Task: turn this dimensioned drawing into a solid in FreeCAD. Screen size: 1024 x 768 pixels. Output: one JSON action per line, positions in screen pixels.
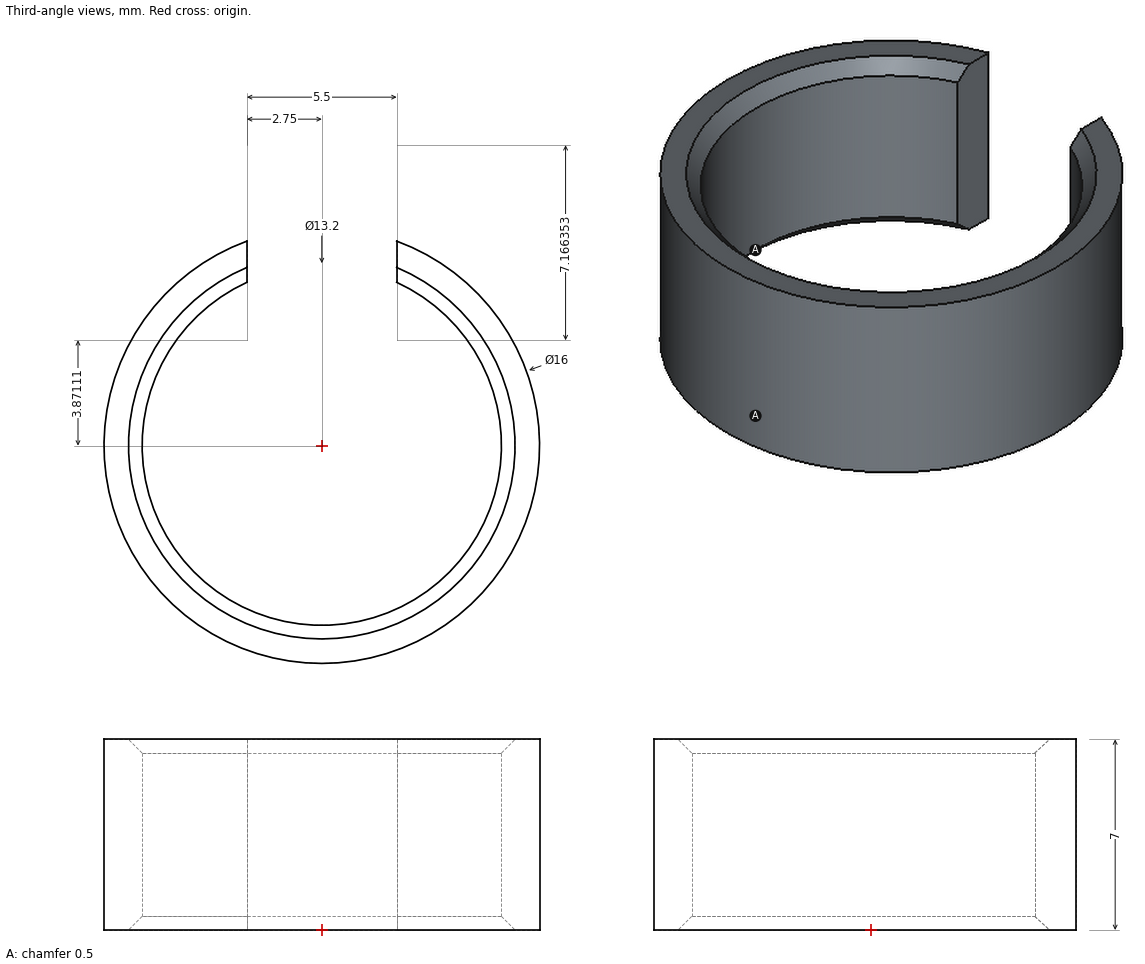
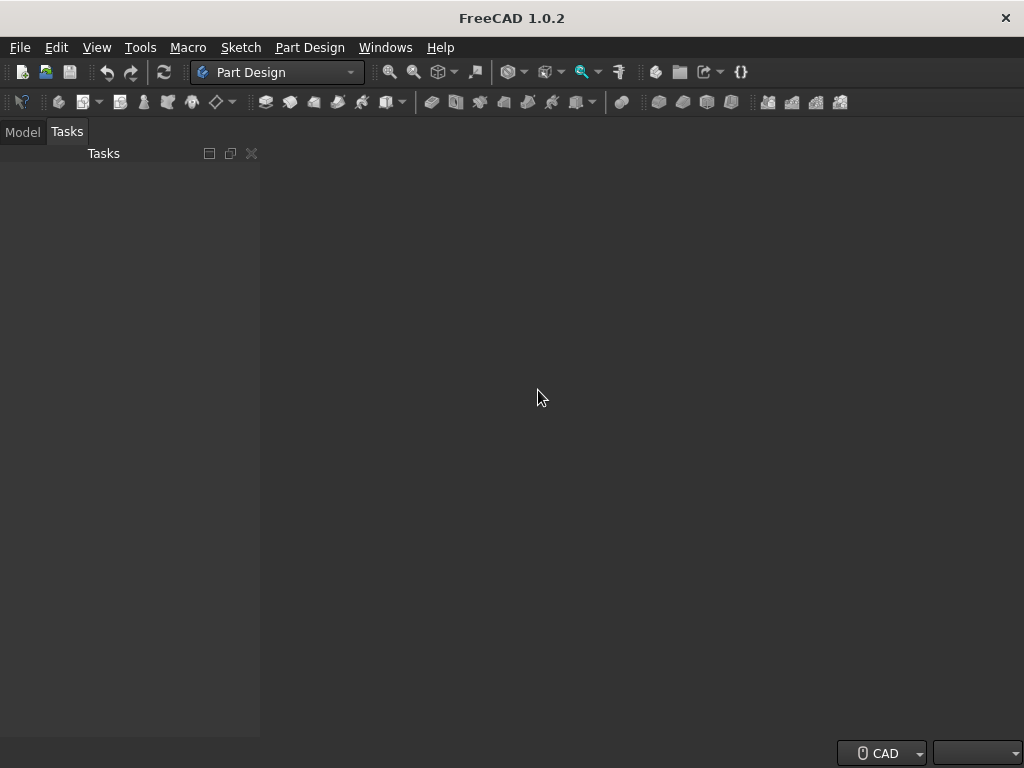
{"action": "left_click", "coordinate": [22, 72]}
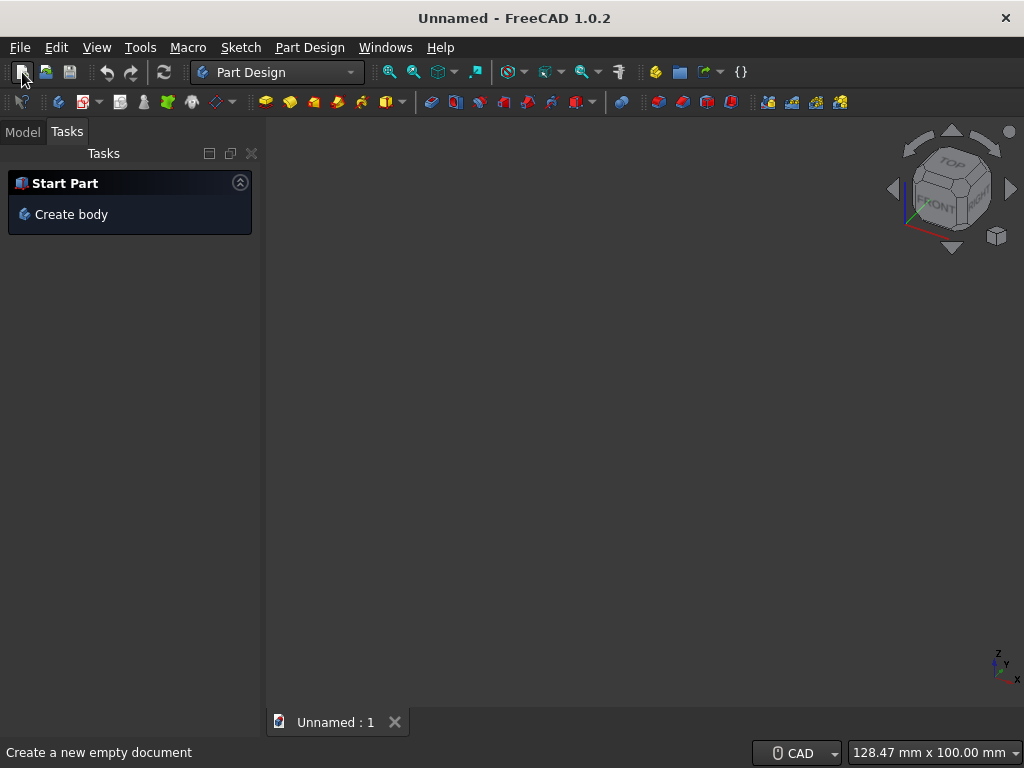
{"action": "left_click", "coordinate": [84, 102]}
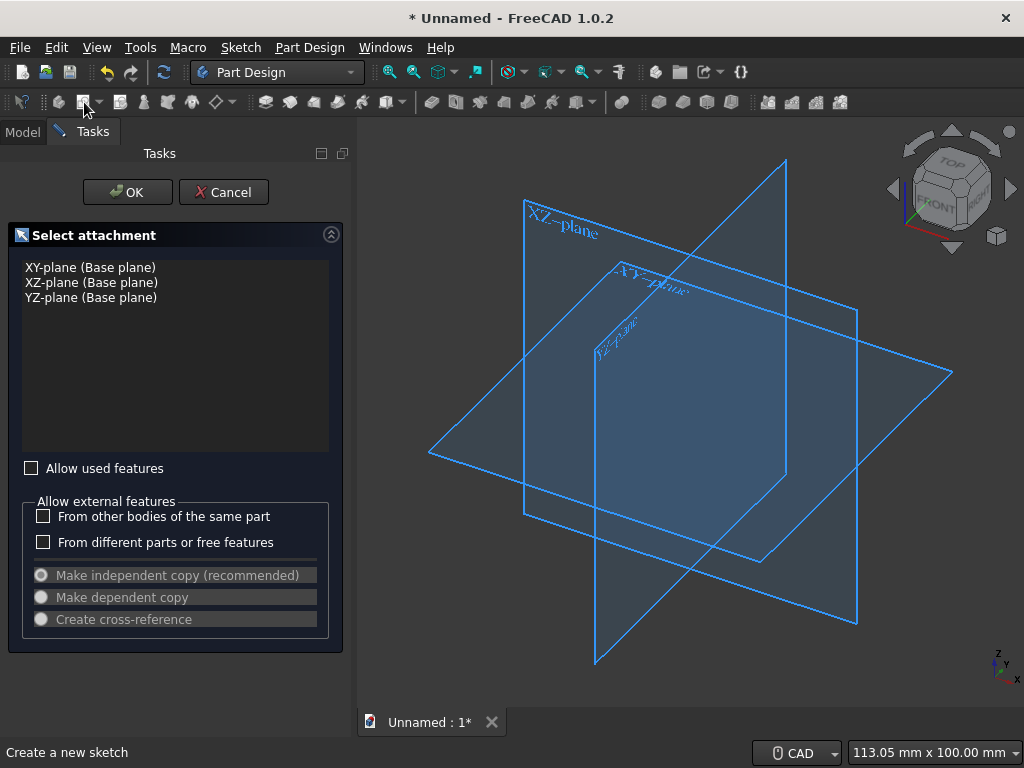
{"action": "left_click", "coordinate": [82, 268]}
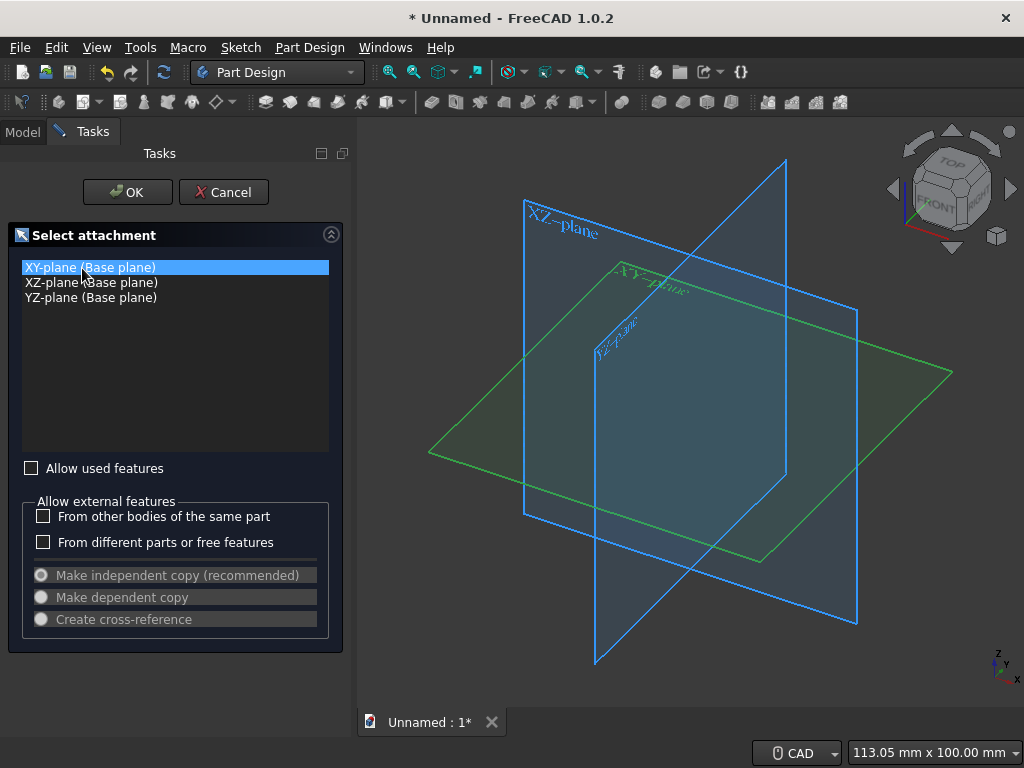
{"action": "left_click", "coordinate": [128, 192]}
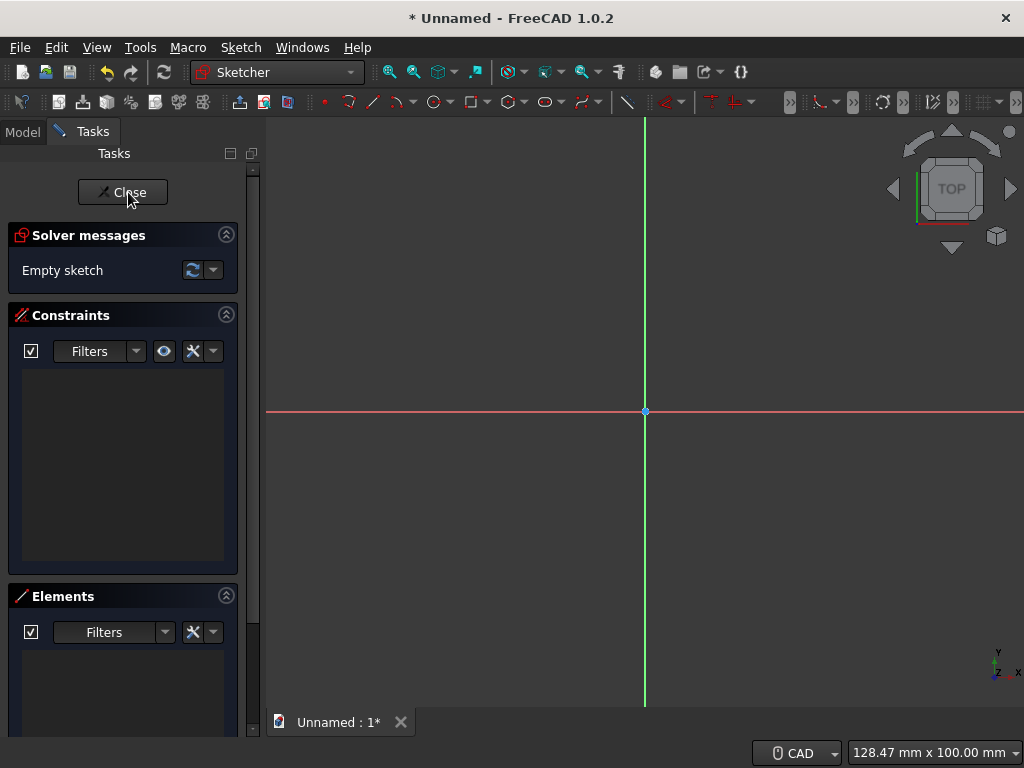
{"action": "scroll", "coordinate": [667, 412], "scroll_direction": "up", "scroll_amount": 7}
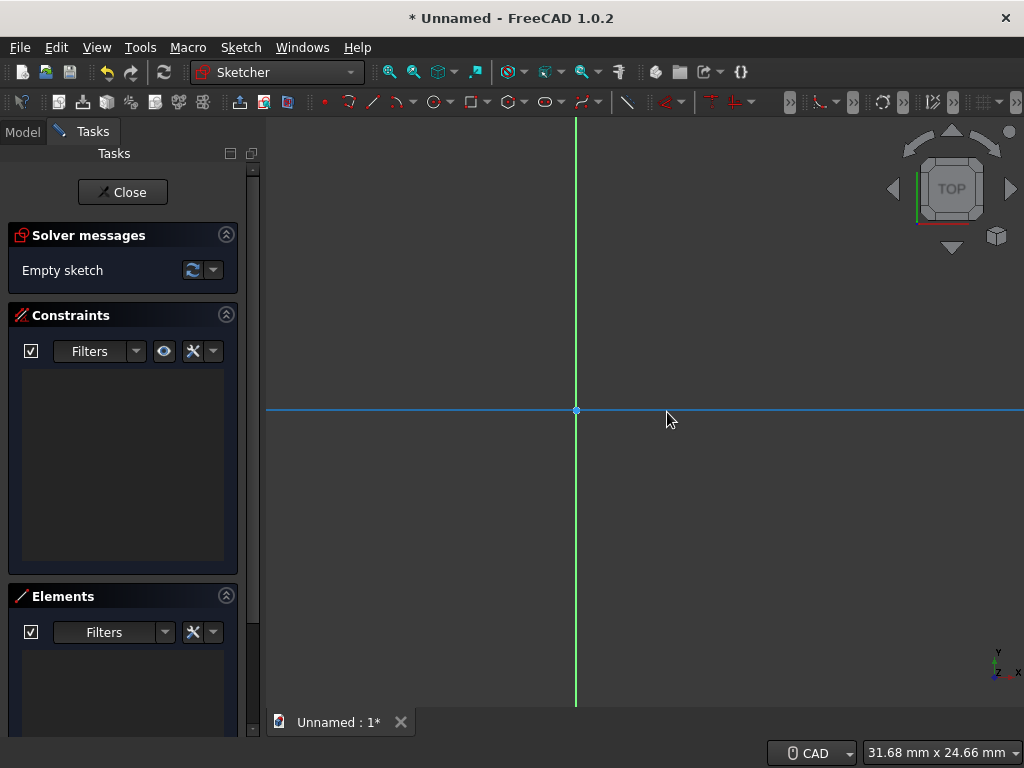
{"action": "left_click", "coordinate": [434, 102]}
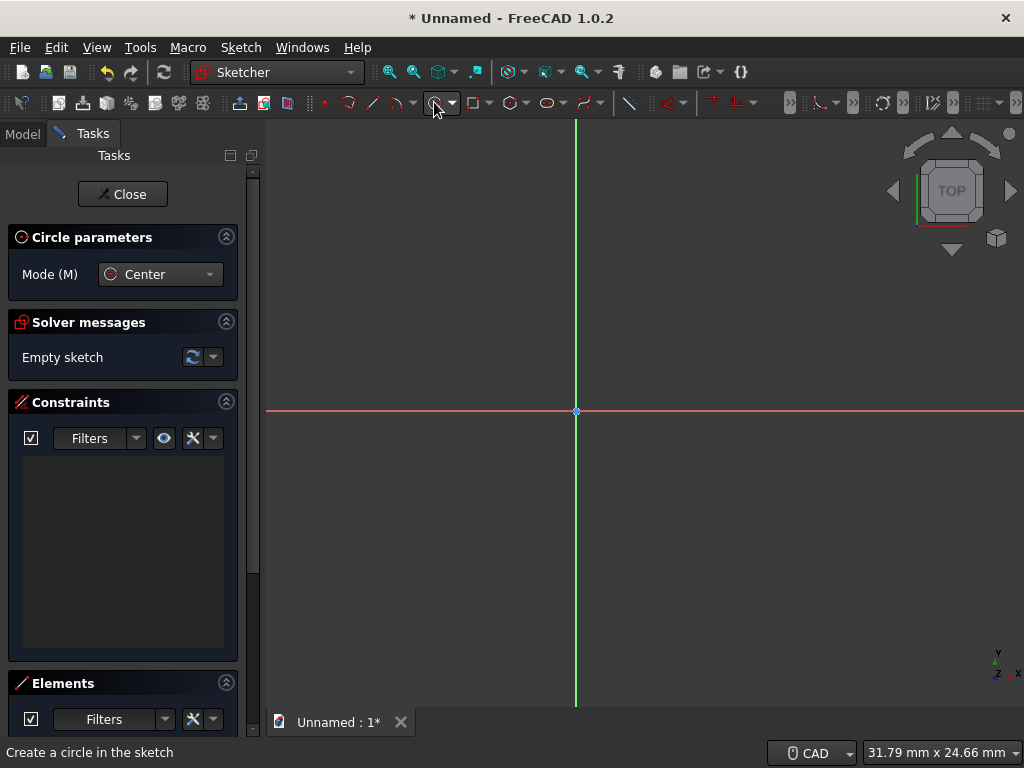
{"action": "left_click", "coordinate": [576, 411]}
{"action": "mouse_move", "coordinate": [711, 277]}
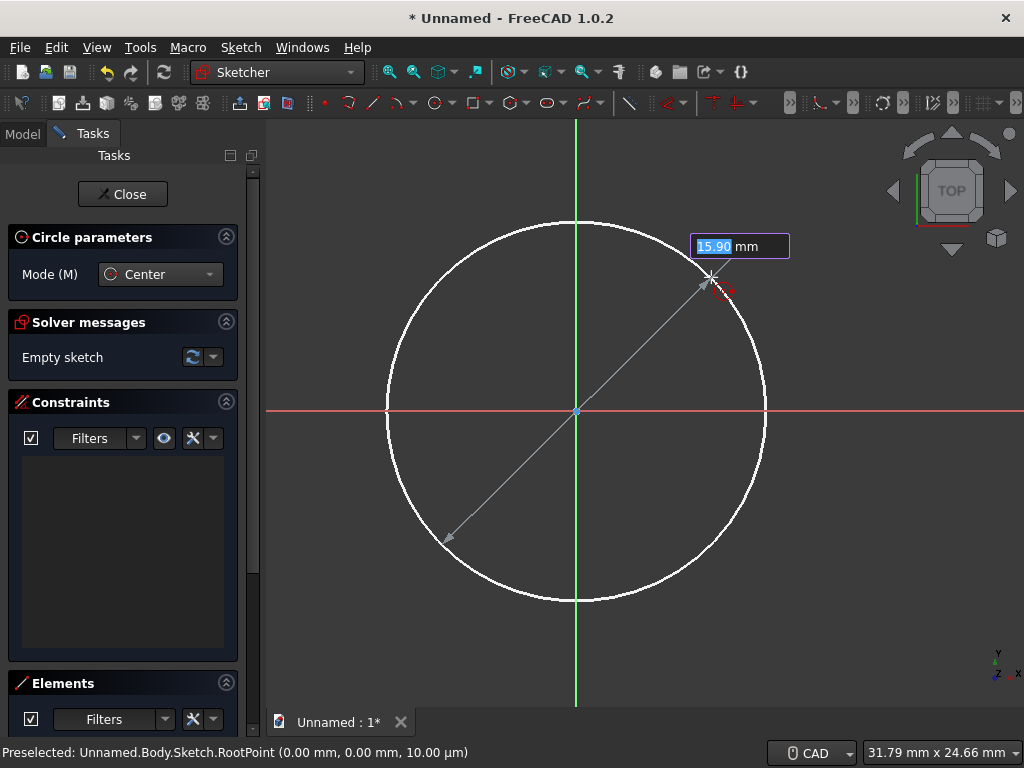
{"action": "type", "text": "16"}
{"action": "key", "text": "Return"}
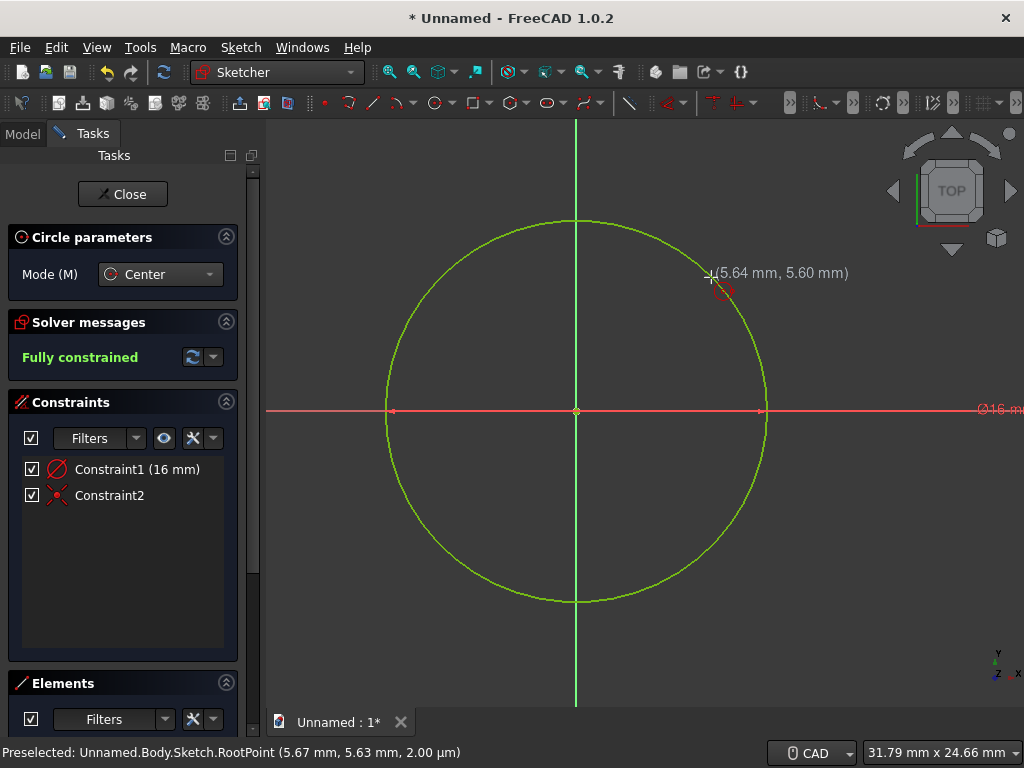
{"action": "left_click", "coordinate": [576, 411]}
{"action": "mouse_move", "coordinate": [688, 300]}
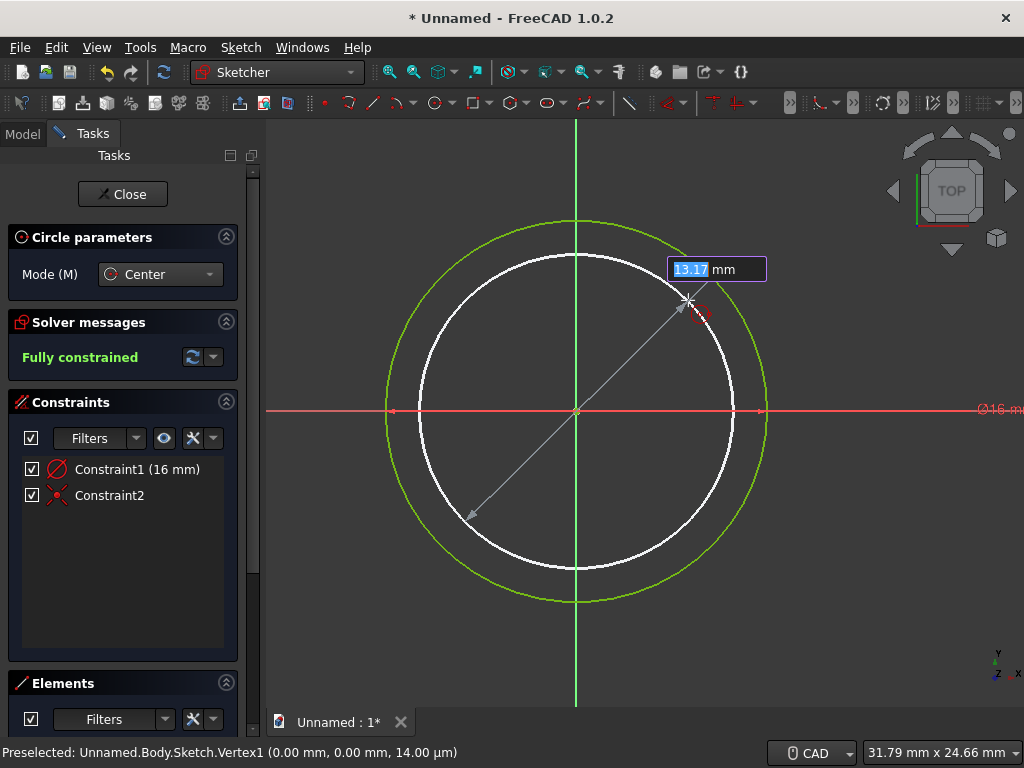
{"action": "type", "text": "13.2"}
{"action": "key", "text": "Return"}
{"action": "key", "text": "Escape"}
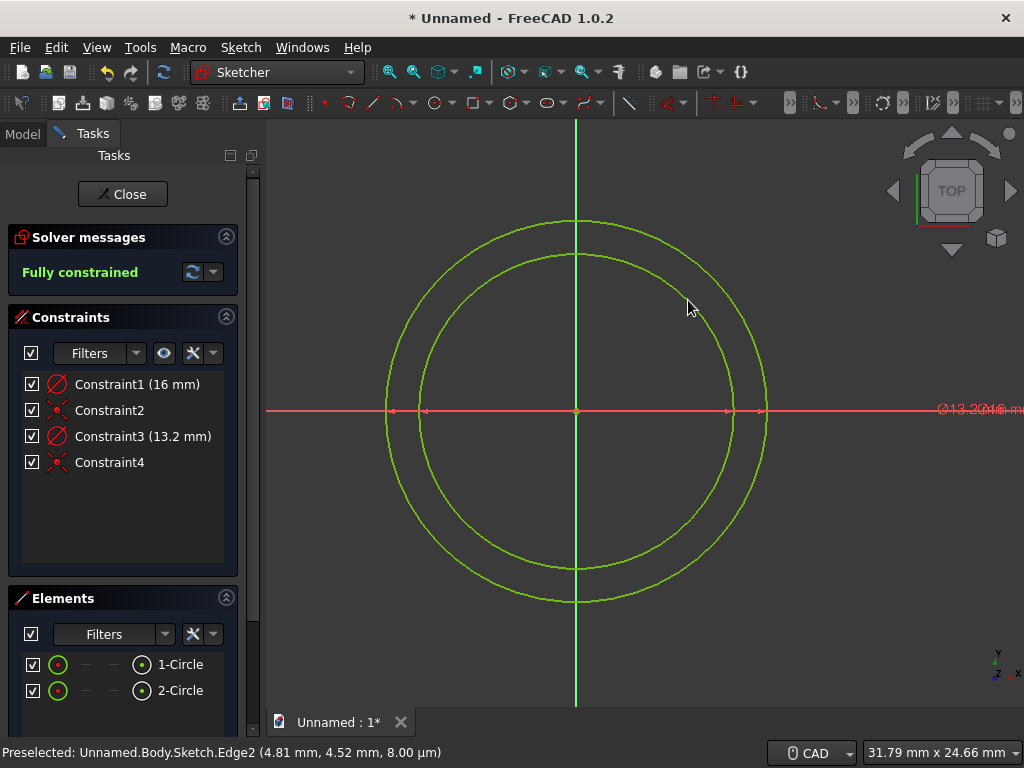
{"action": "left_click", "coordinate": [123, 194]}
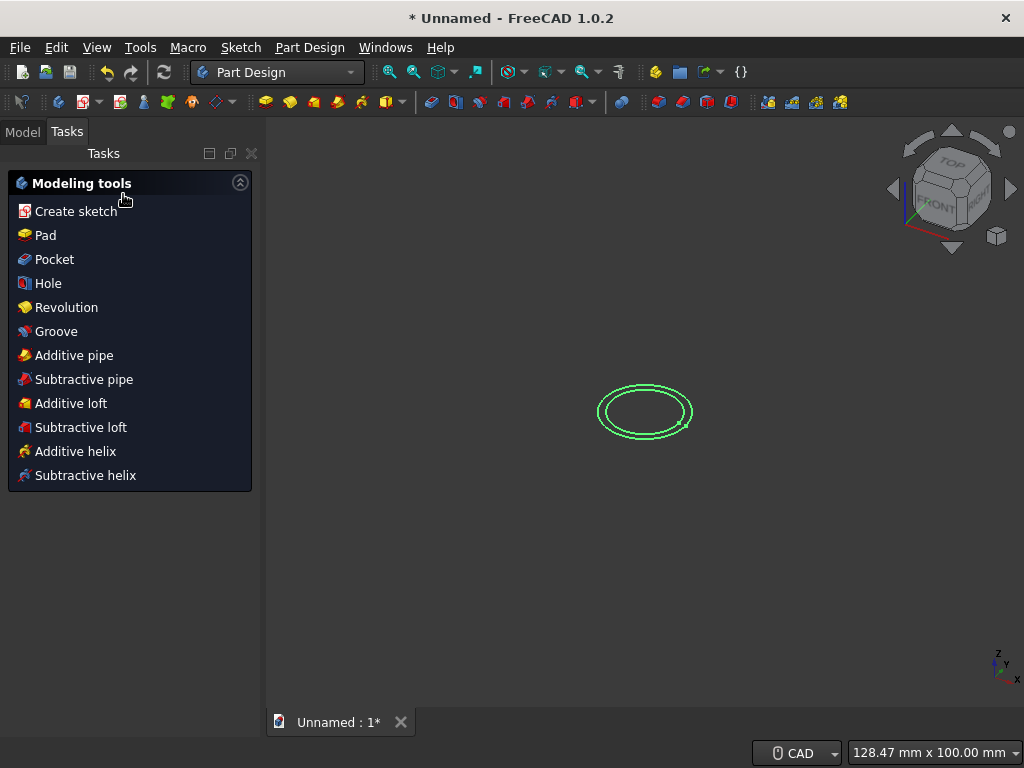
{"action": "left_click", "coordinate": [266, 102]}